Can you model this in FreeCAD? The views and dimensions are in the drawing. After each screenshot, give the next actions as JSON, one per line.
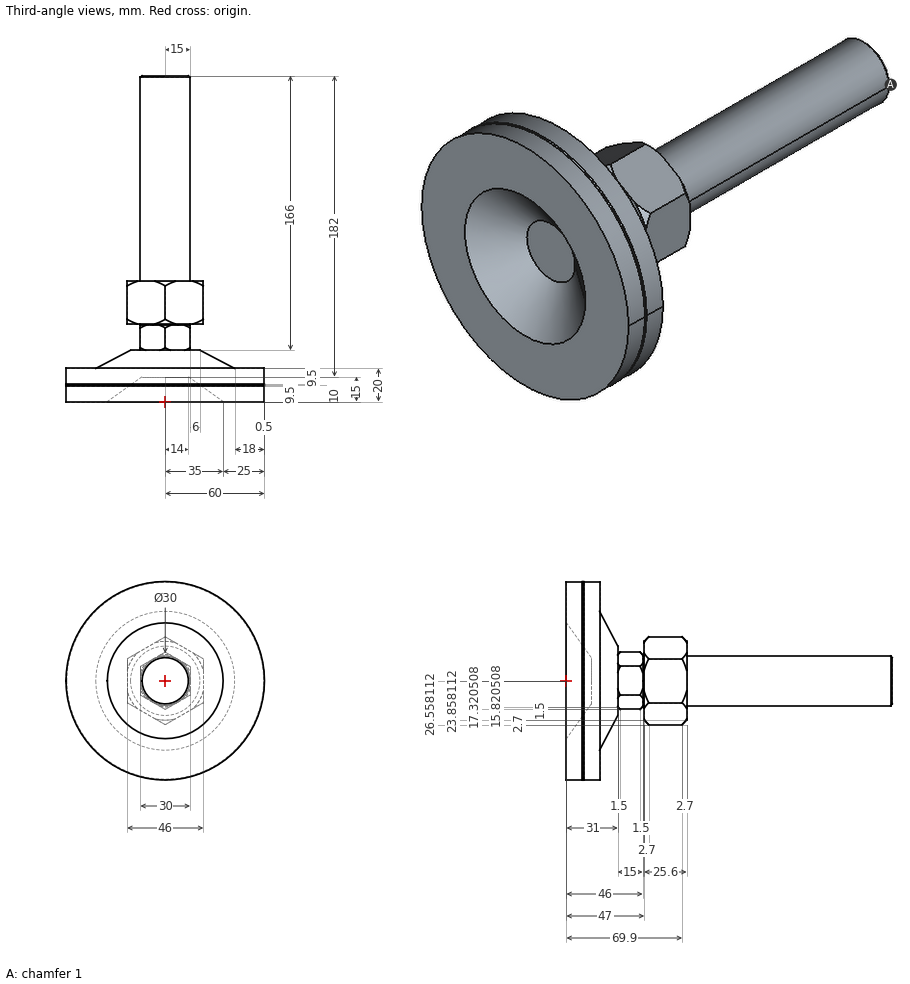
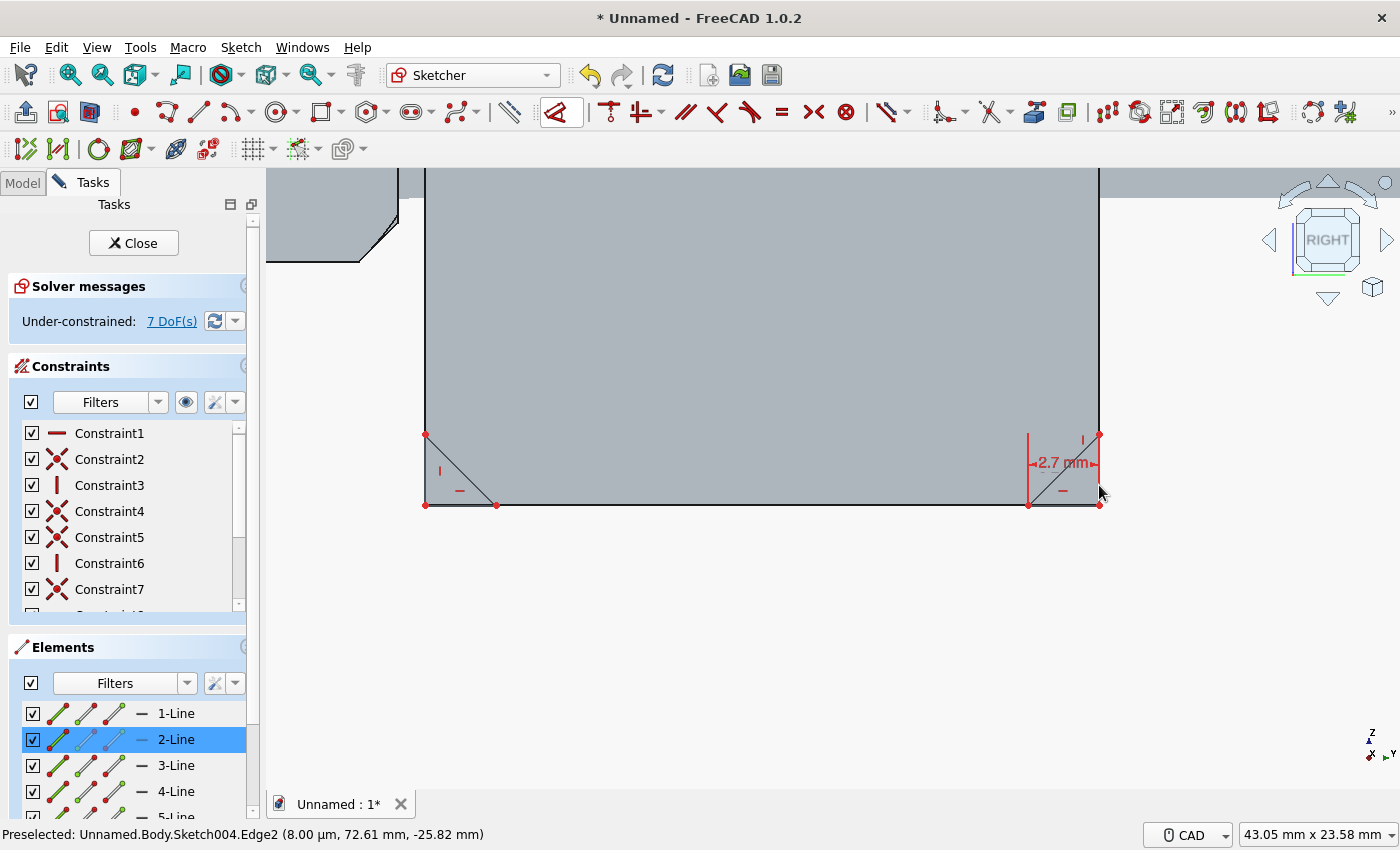
{"action": "key", "text": "i"}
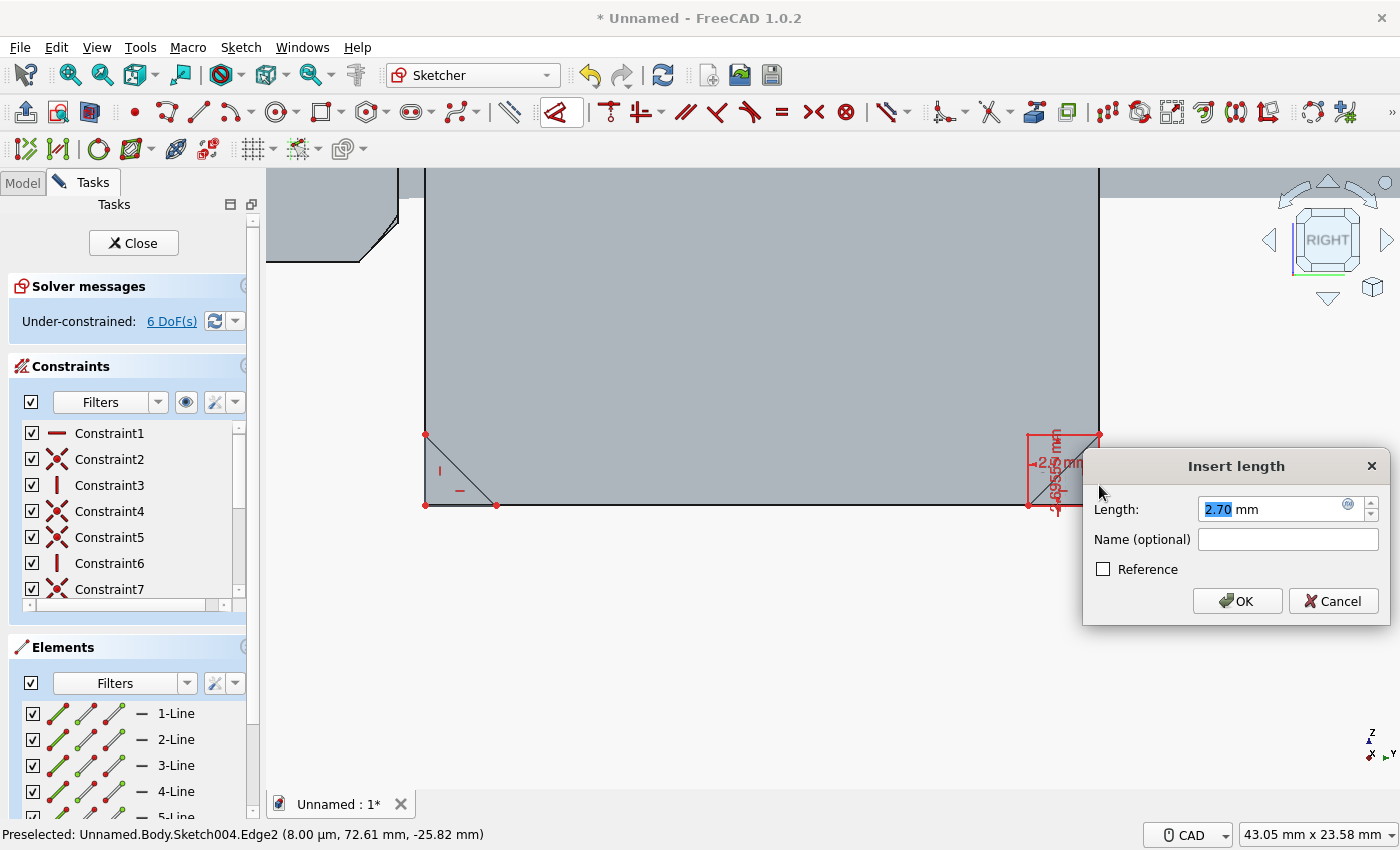
{"action": "type", "text": "2.7"}
{"action": "key", "text": "Return"}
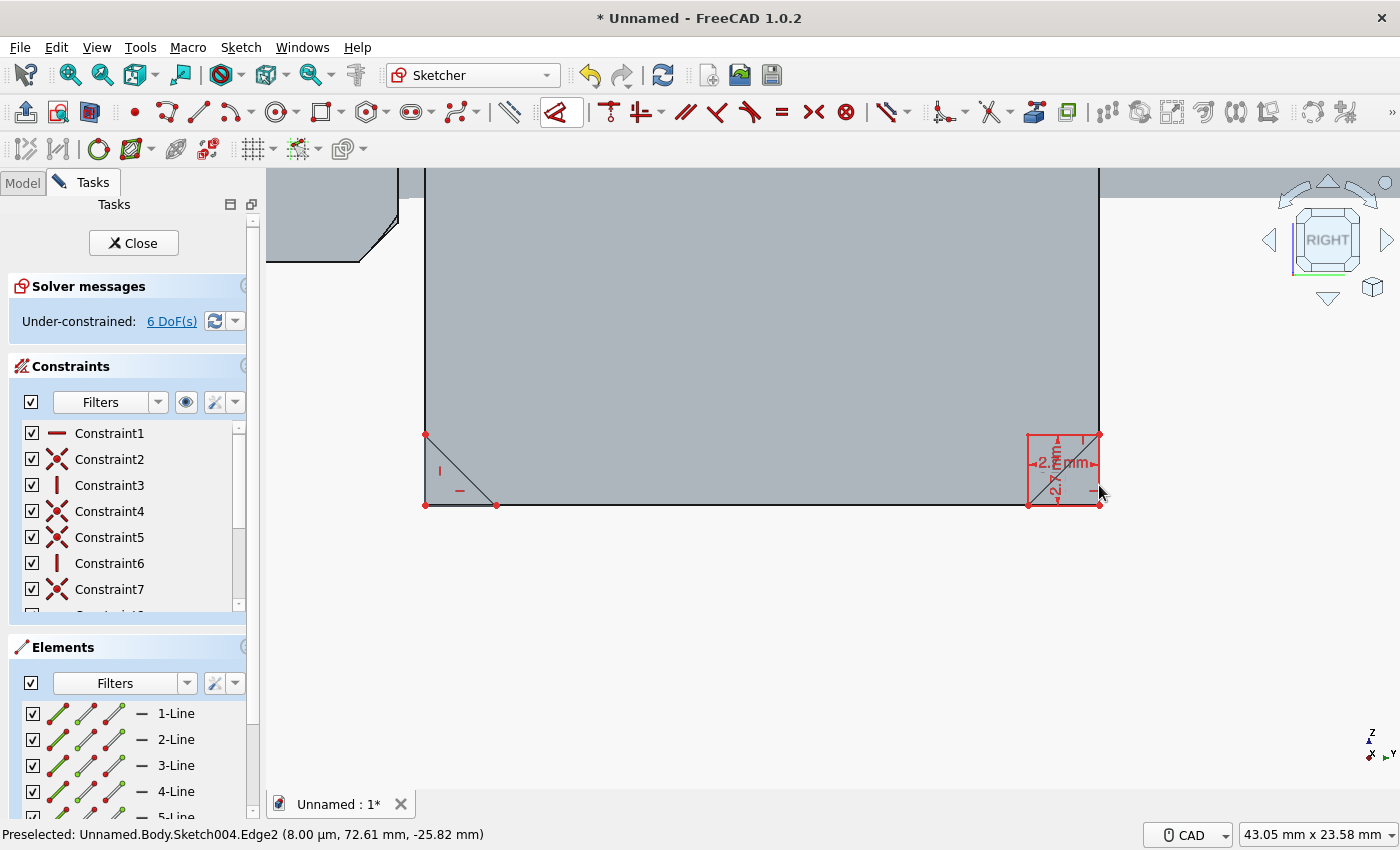
{"action": "left_click", "coordinate": [425, 456]}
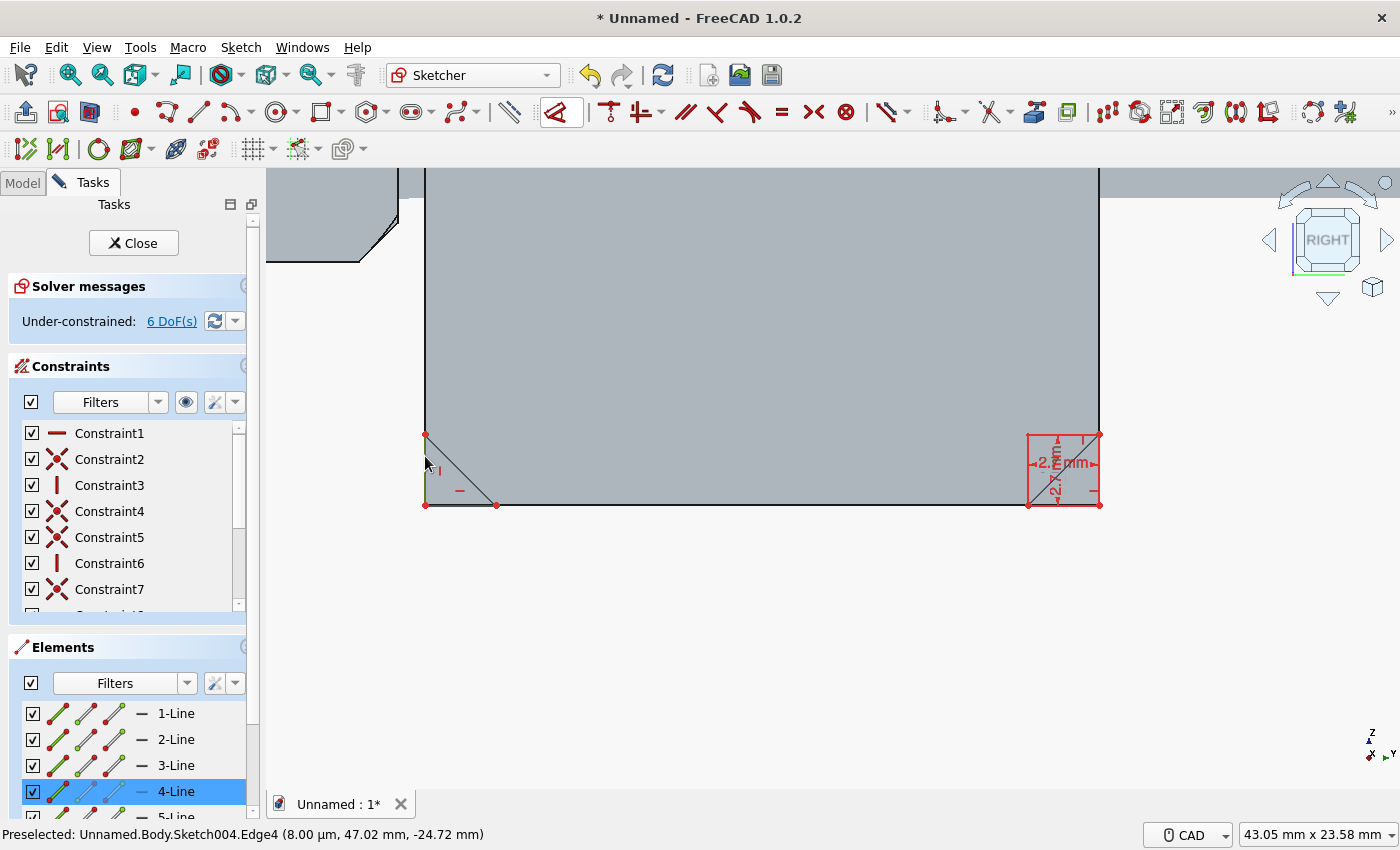
{"action": "key", "text": "i"}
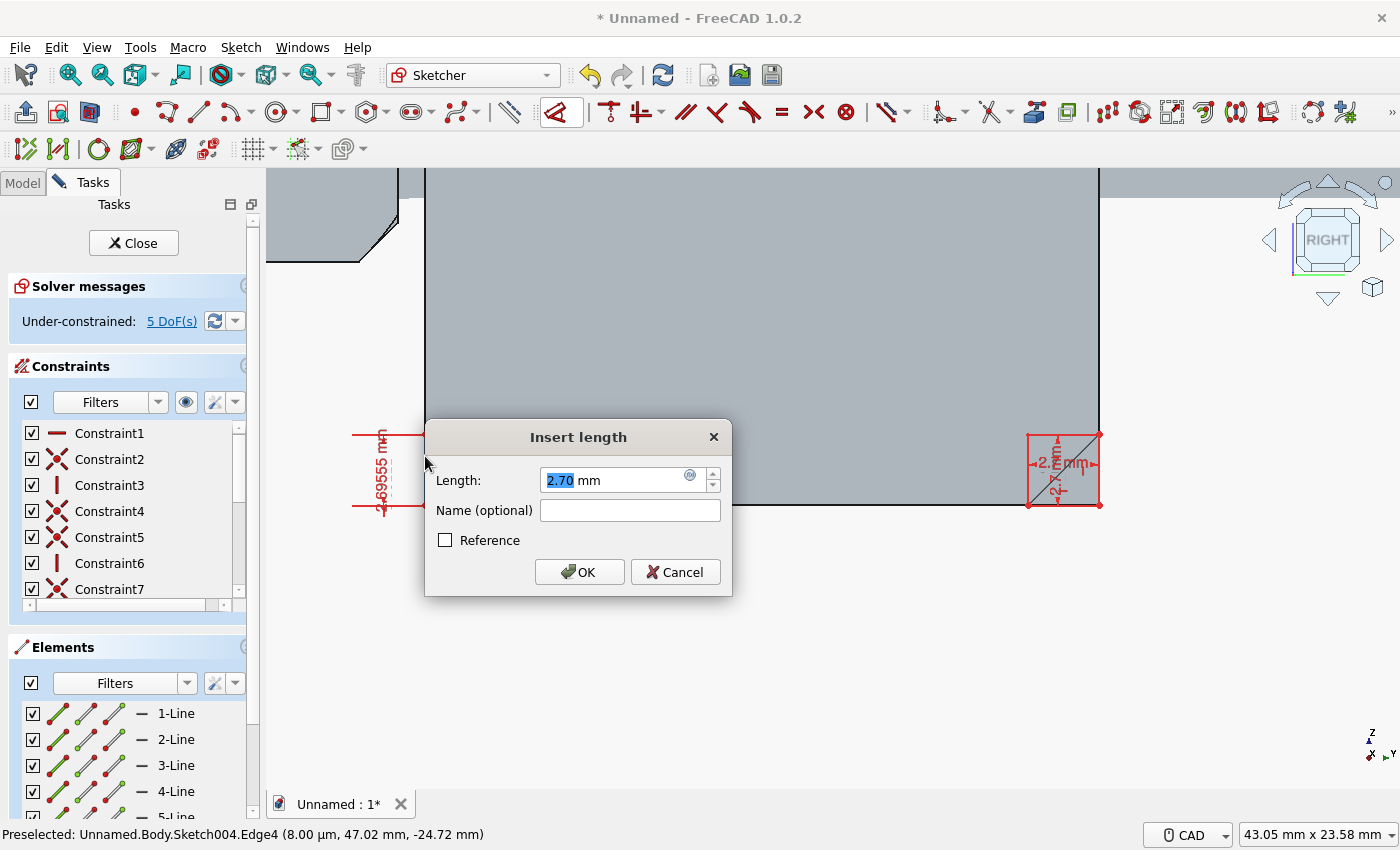
{"action": "type", "text": "2.7"}
{"action": "key", "text": "Return"}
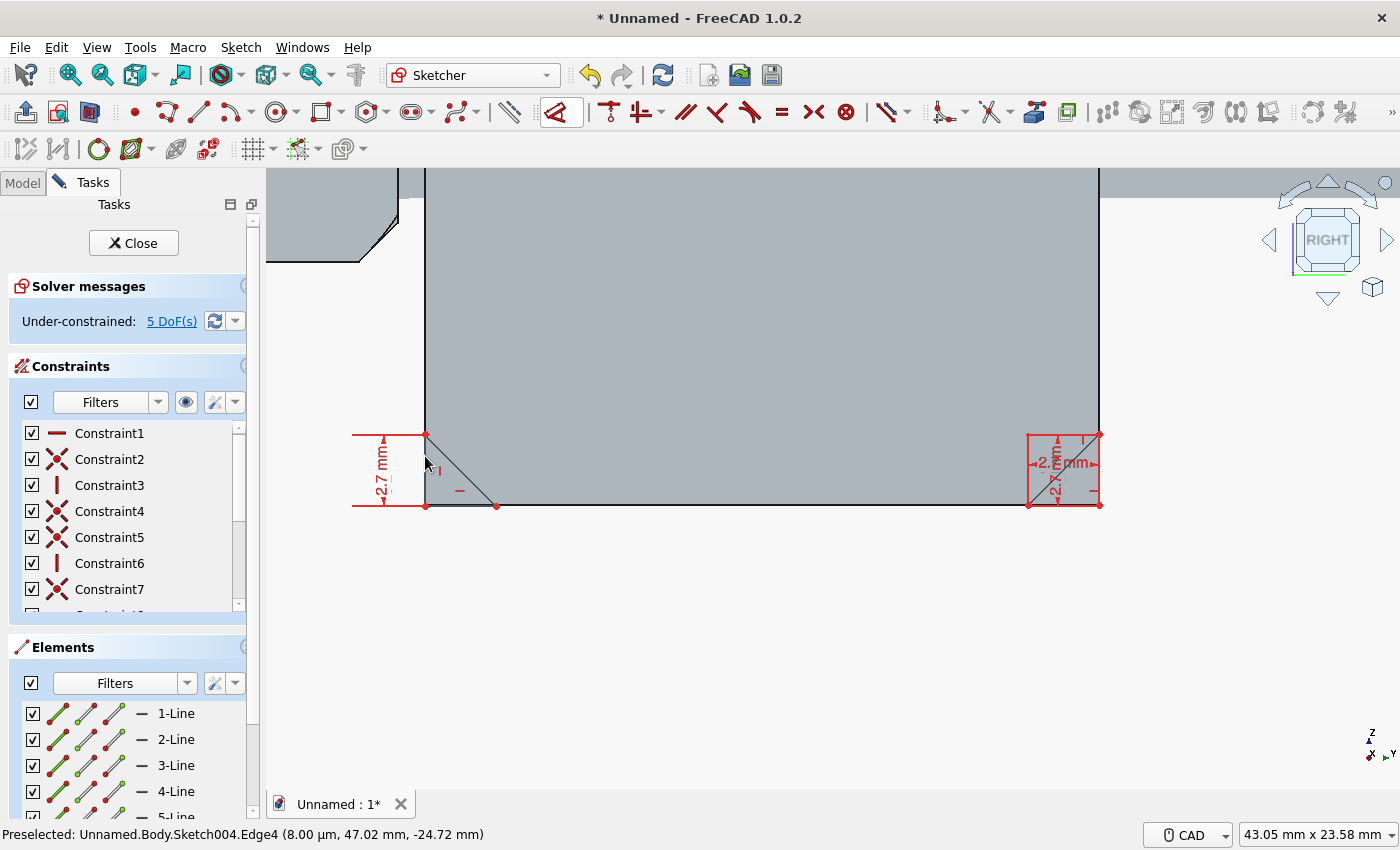
{"action": "left_click", "coordinate": [446, 506]}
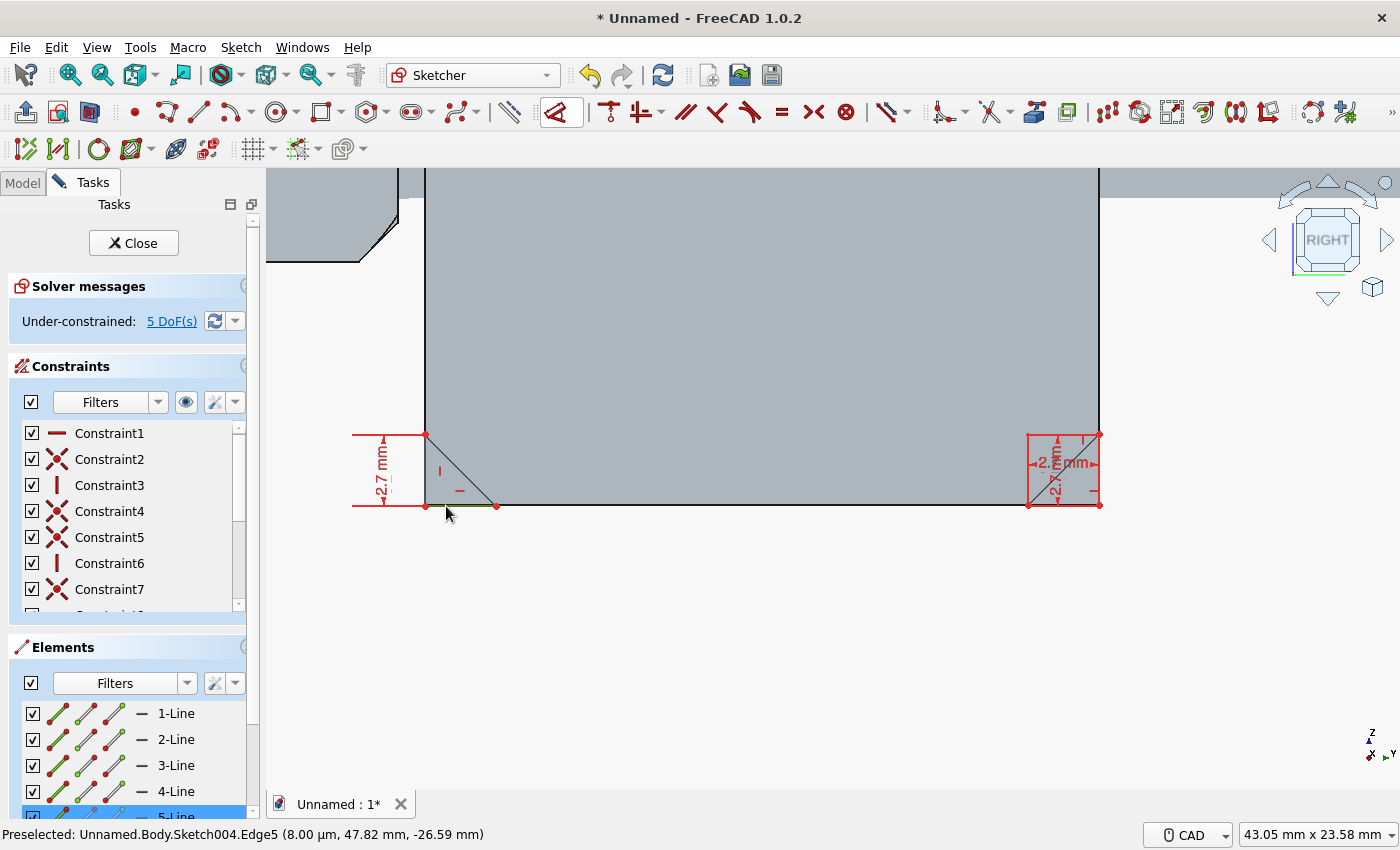
{"action": "key", "text": "l"}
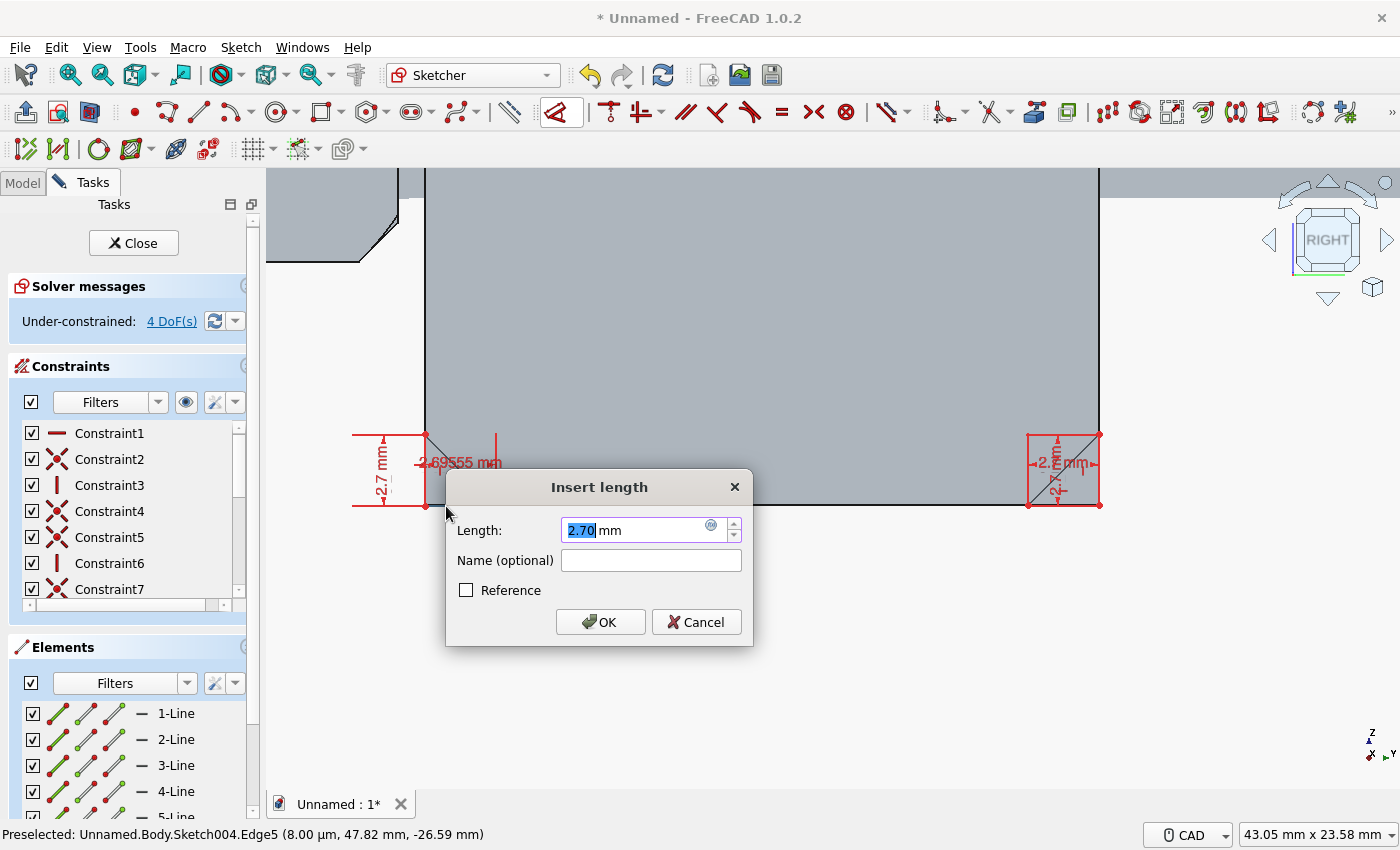
{"action": "type", "text": "2.7"}
{"action": "key", "text": "Return"}